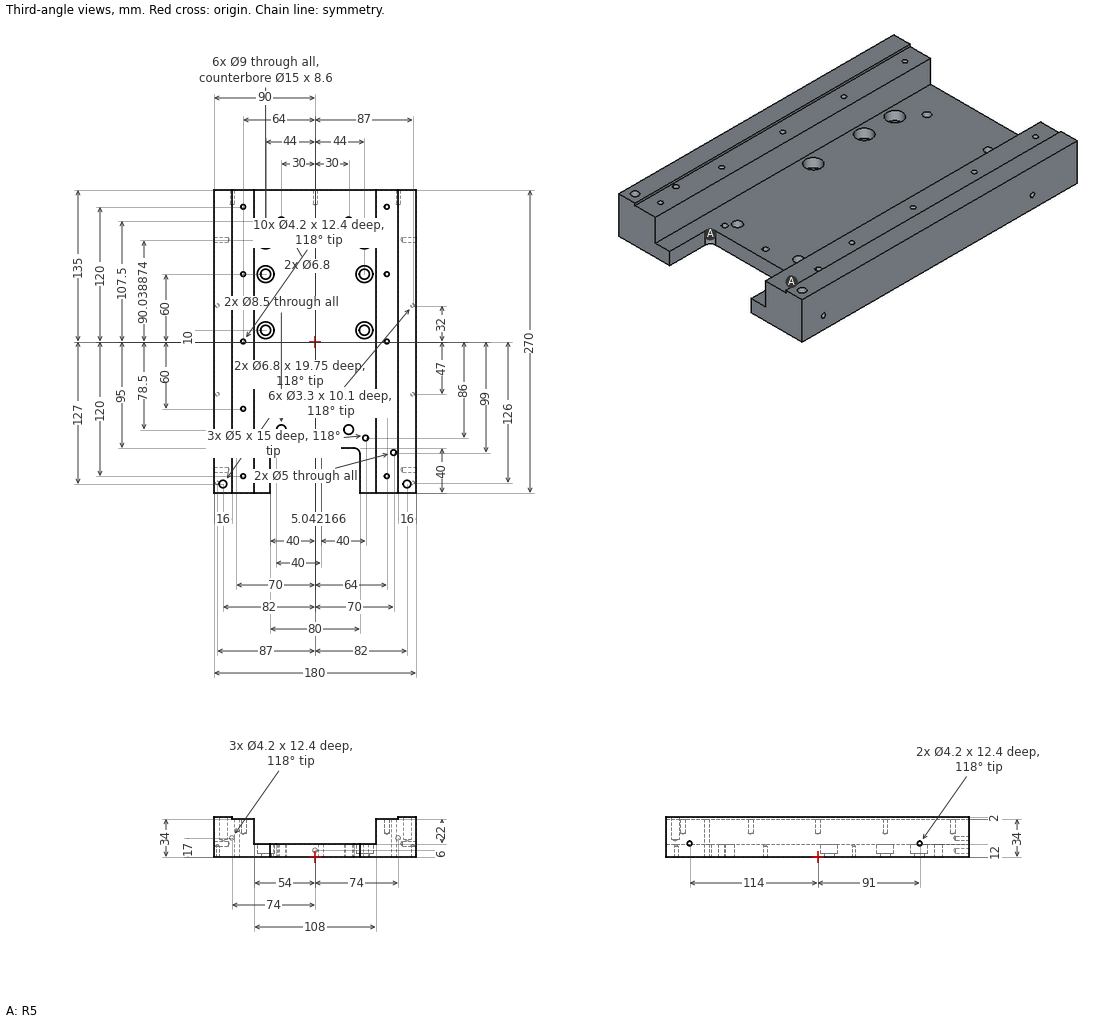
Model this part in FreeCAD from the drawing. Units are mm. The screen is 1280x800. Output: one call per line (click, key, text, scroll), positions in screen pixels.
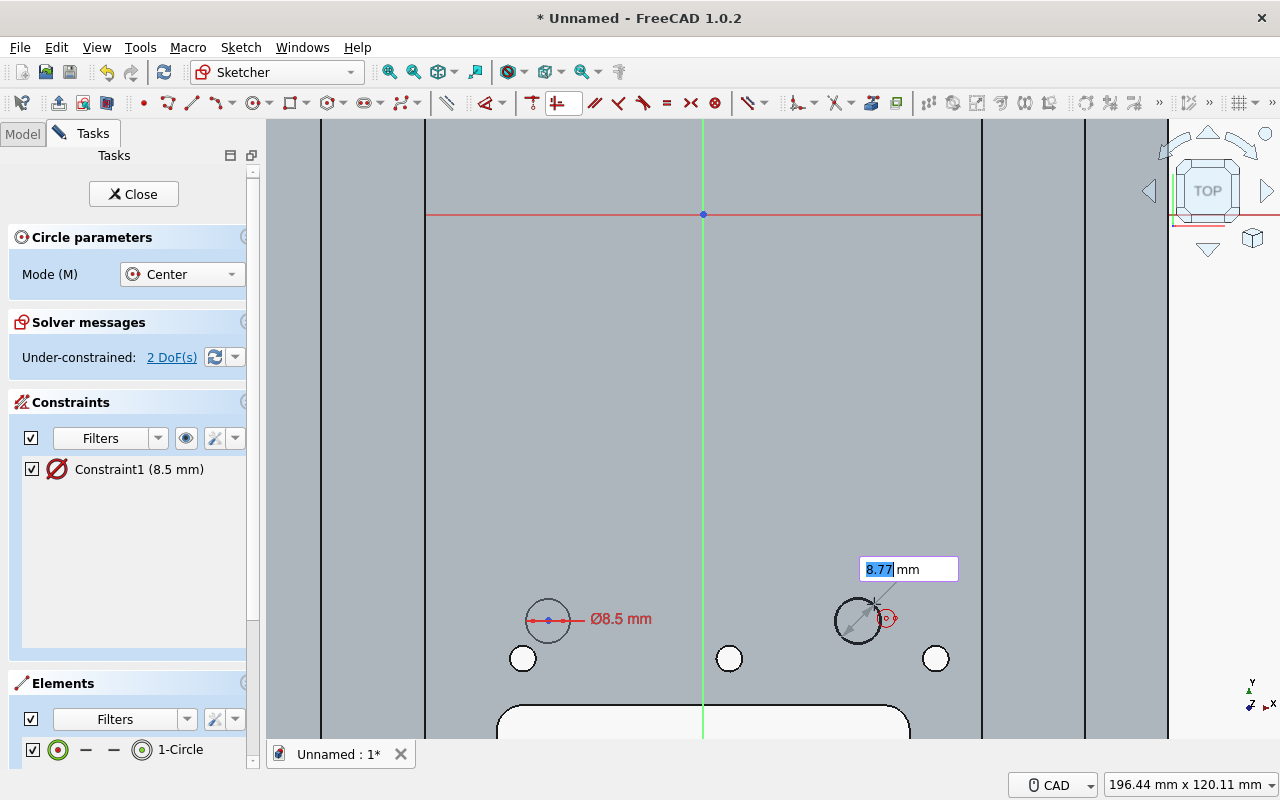
text(8.5)
key(Return)
key(Escape)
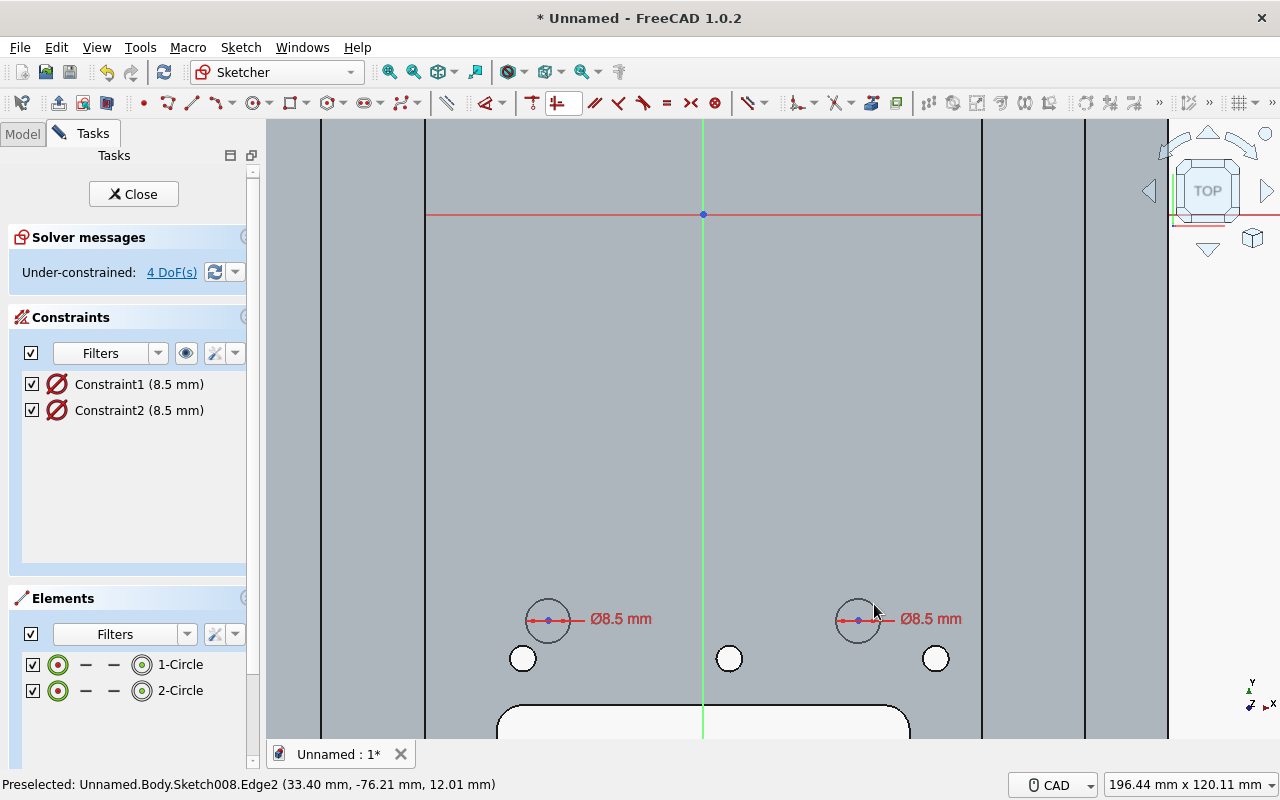
click(548, 621)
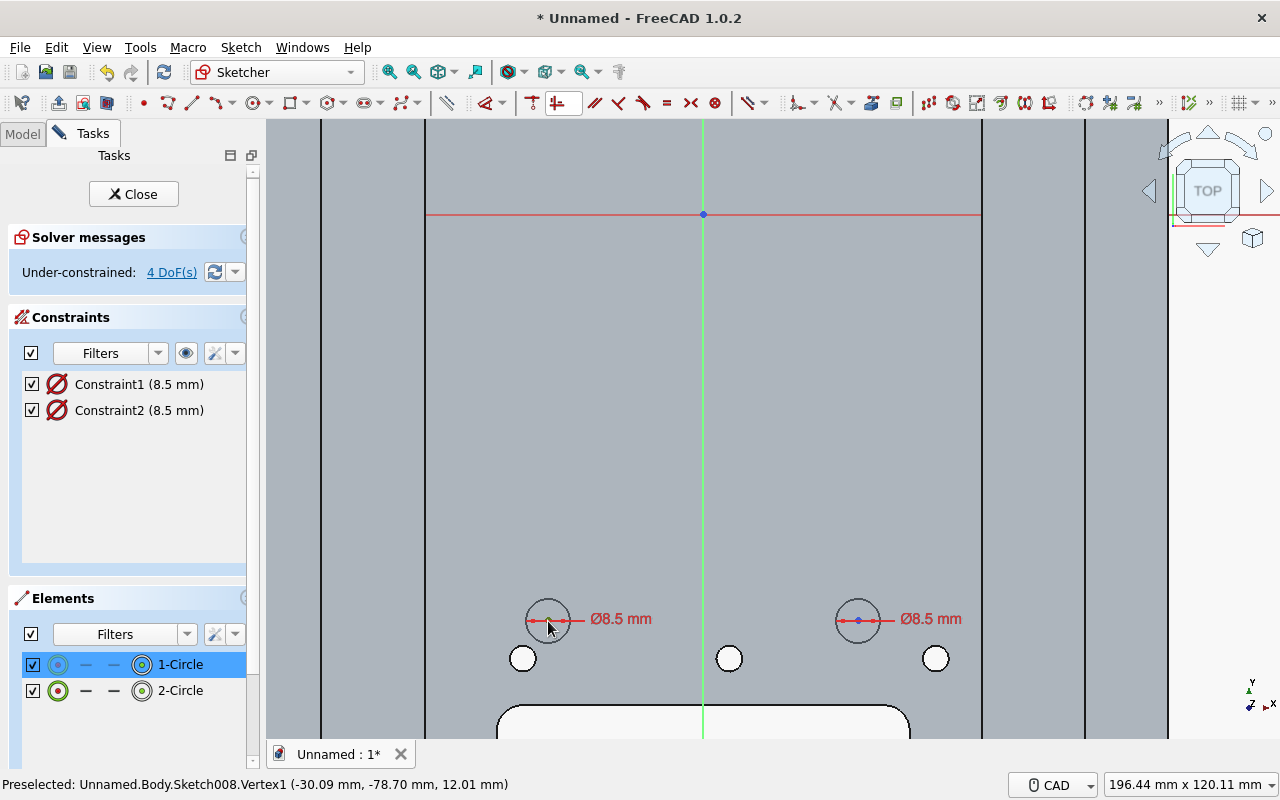
click(858, 621)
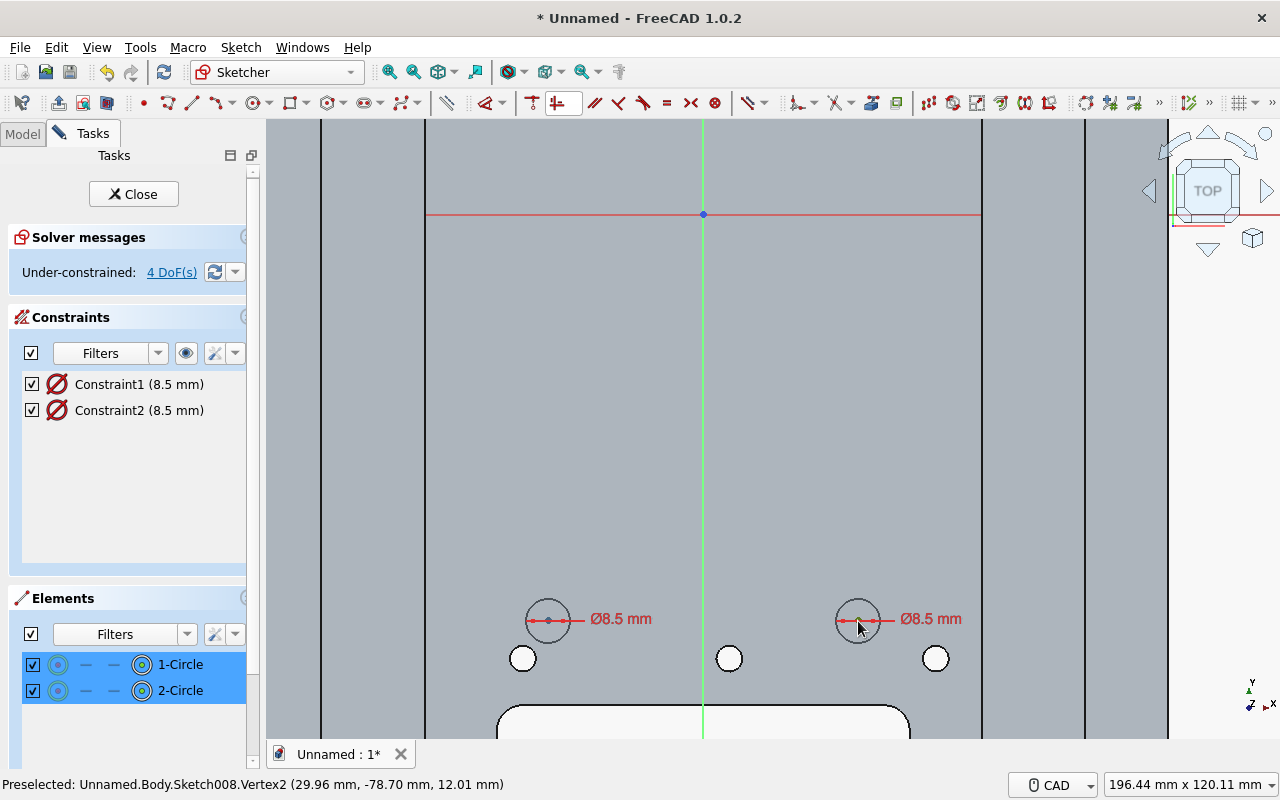
click(576, 104)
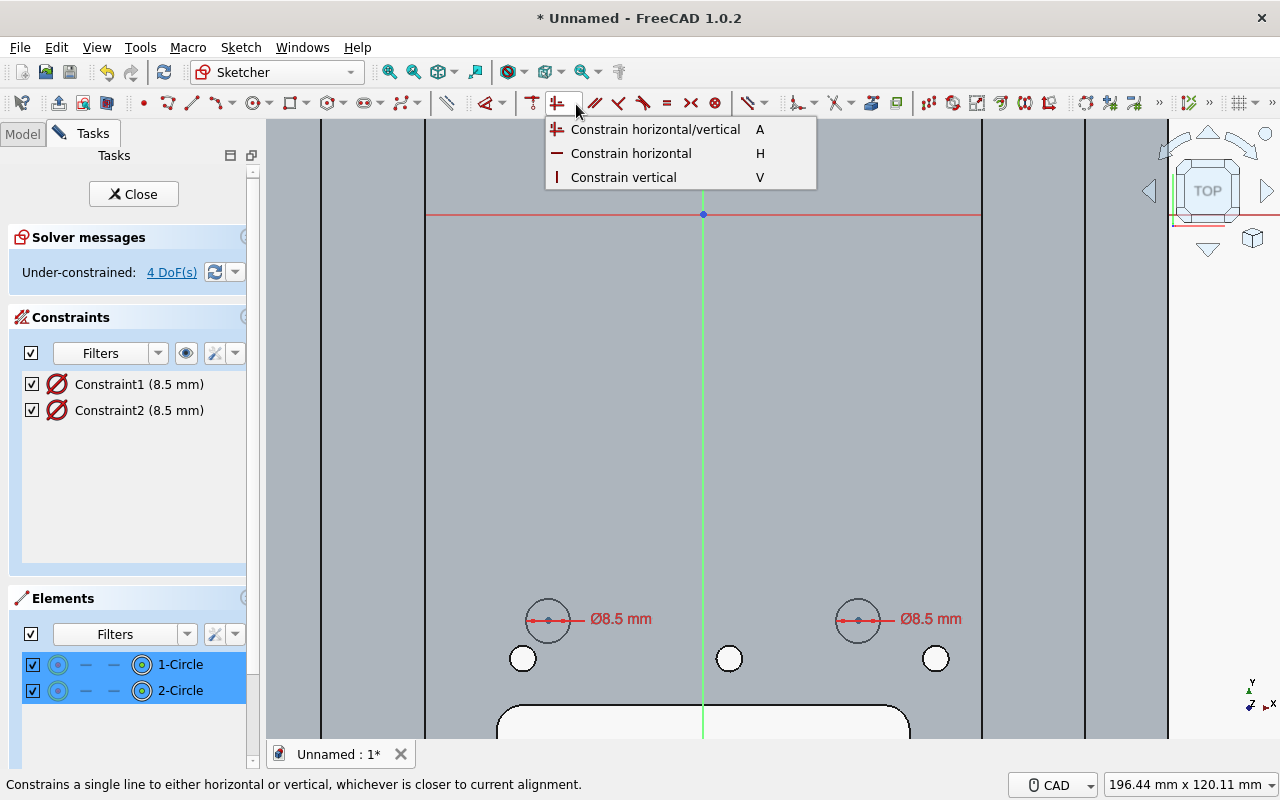
click(681, 153)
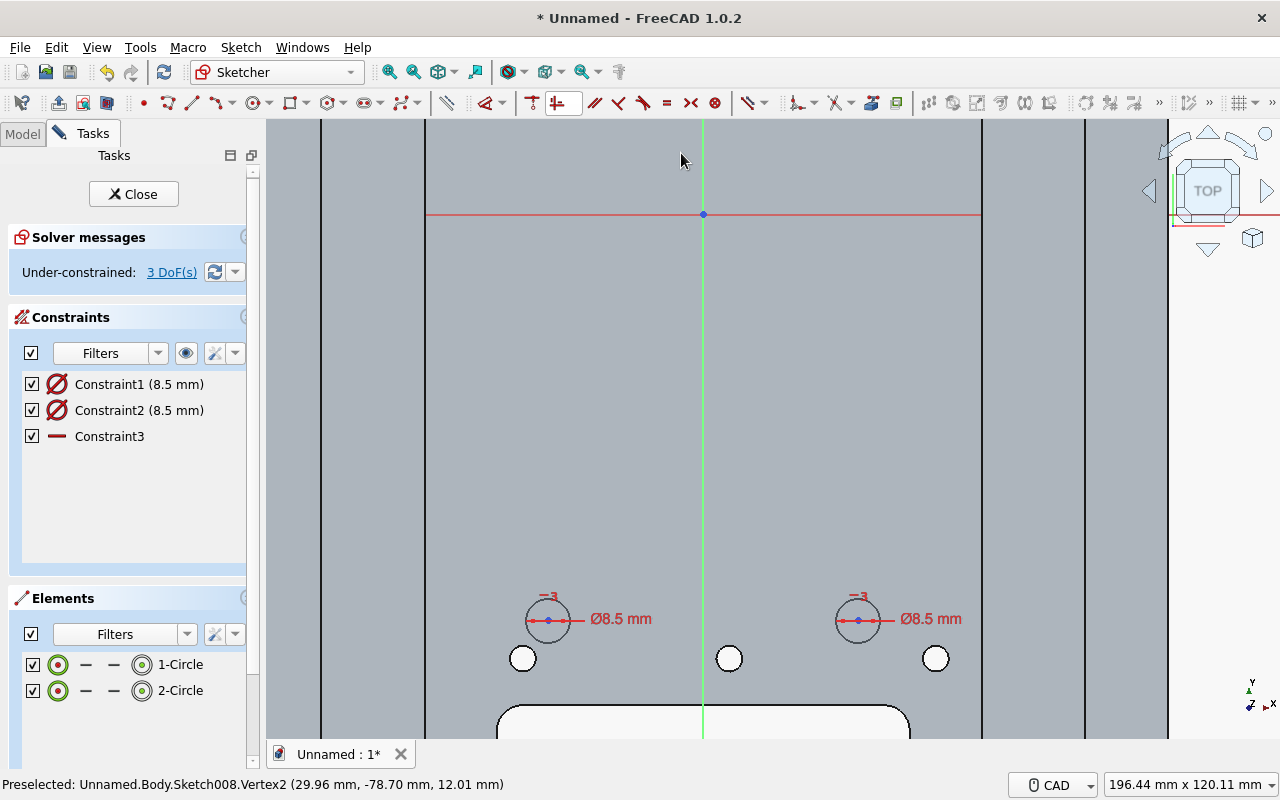
click(486, 104)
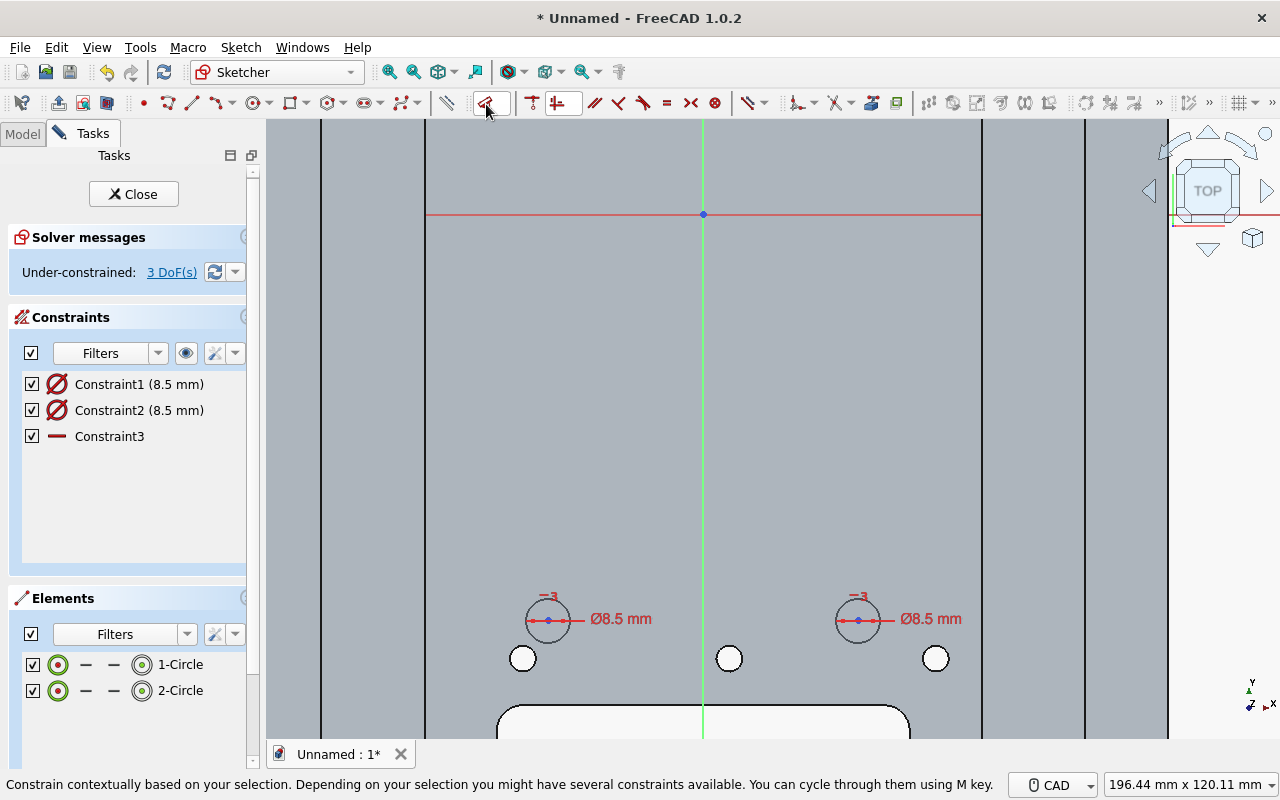
click(548, 621)
click(626, 181)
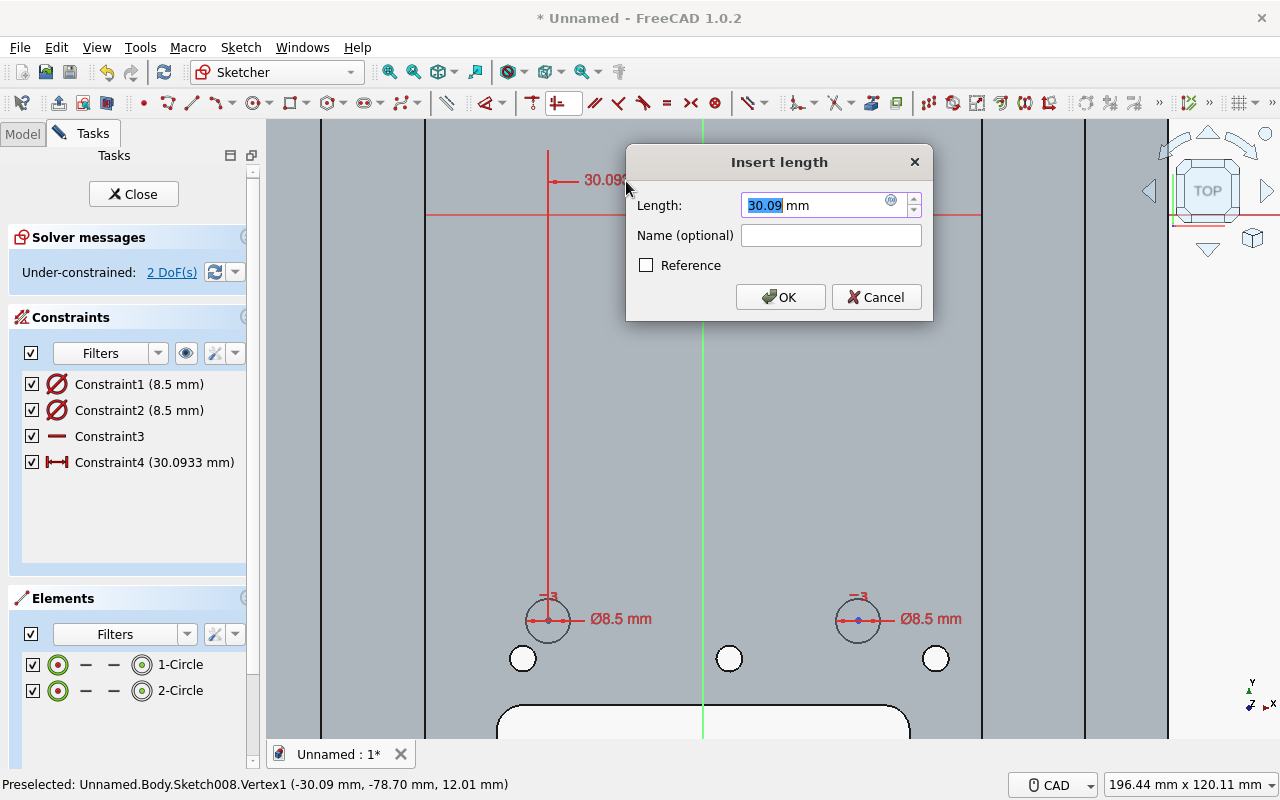
text(30)
key(Return)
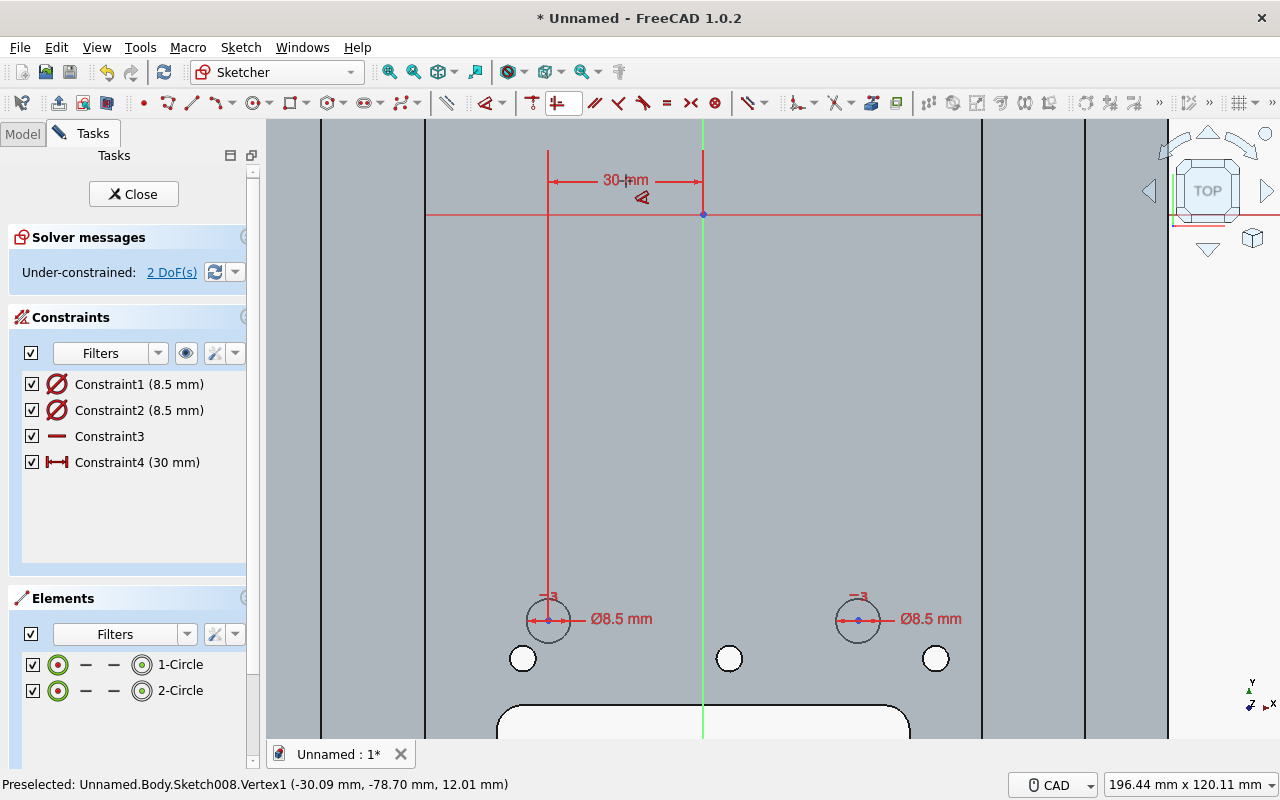
click(858, 621)
click(781, 181)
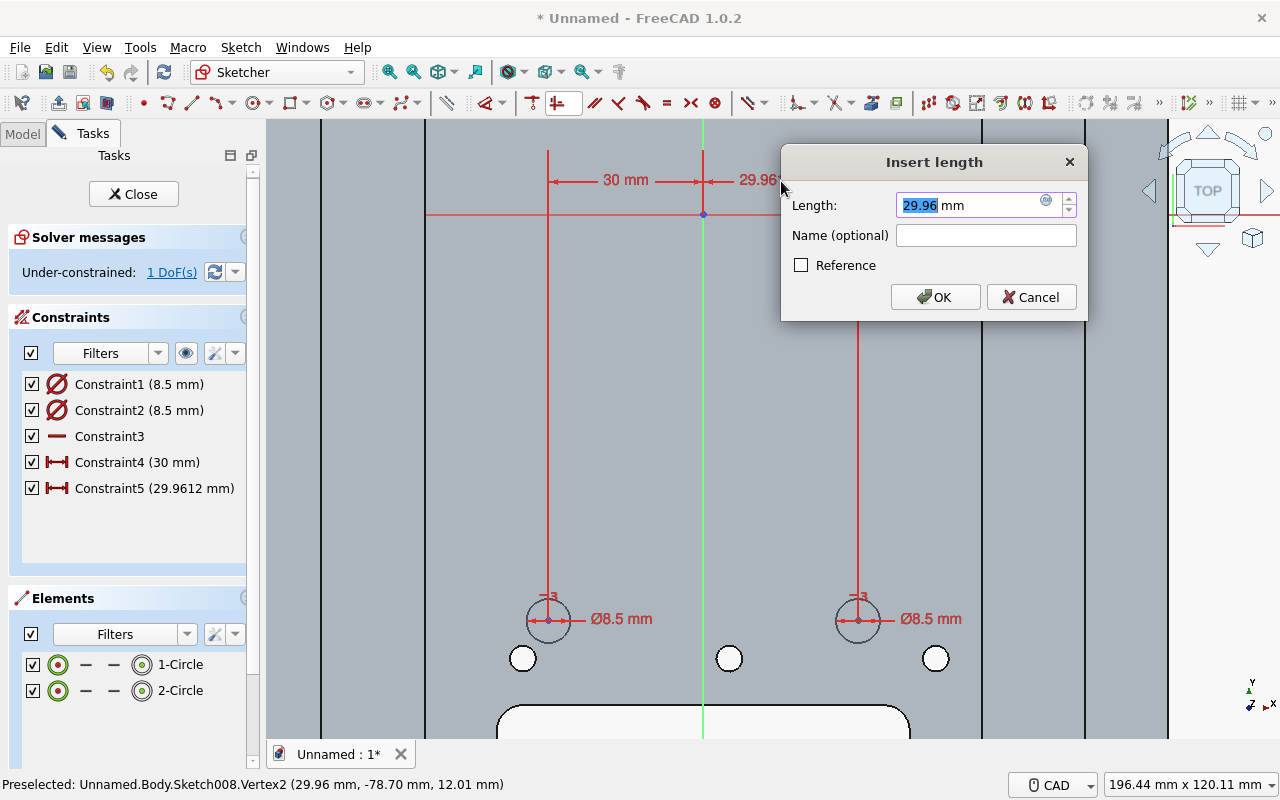
text(30)
key(Return)